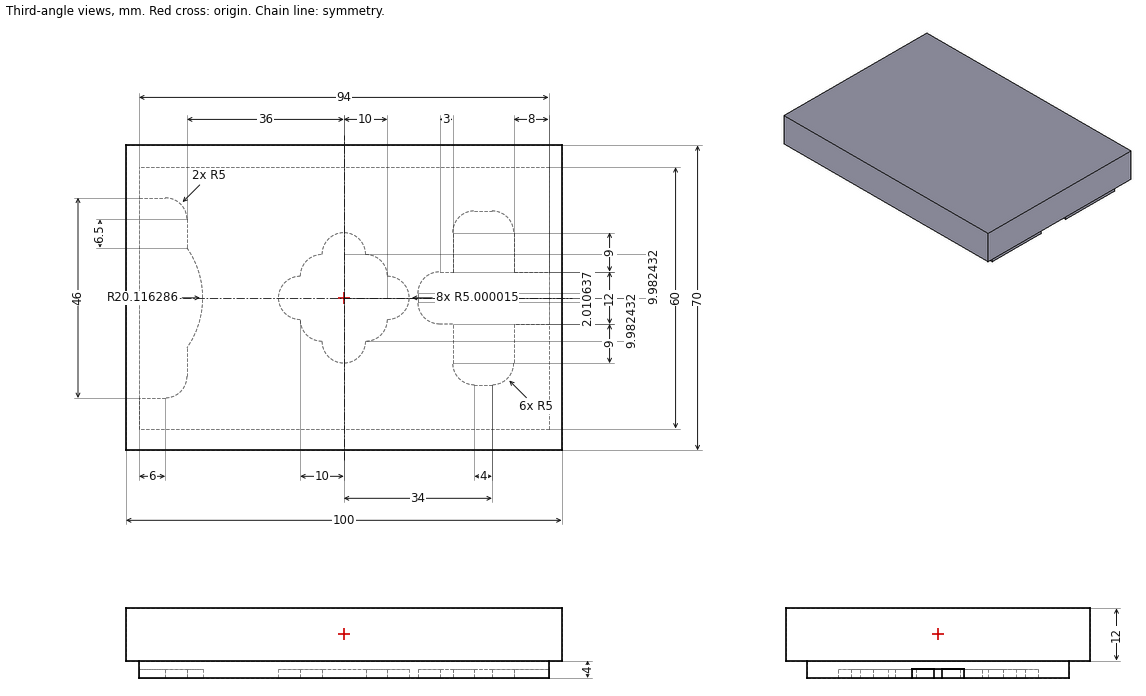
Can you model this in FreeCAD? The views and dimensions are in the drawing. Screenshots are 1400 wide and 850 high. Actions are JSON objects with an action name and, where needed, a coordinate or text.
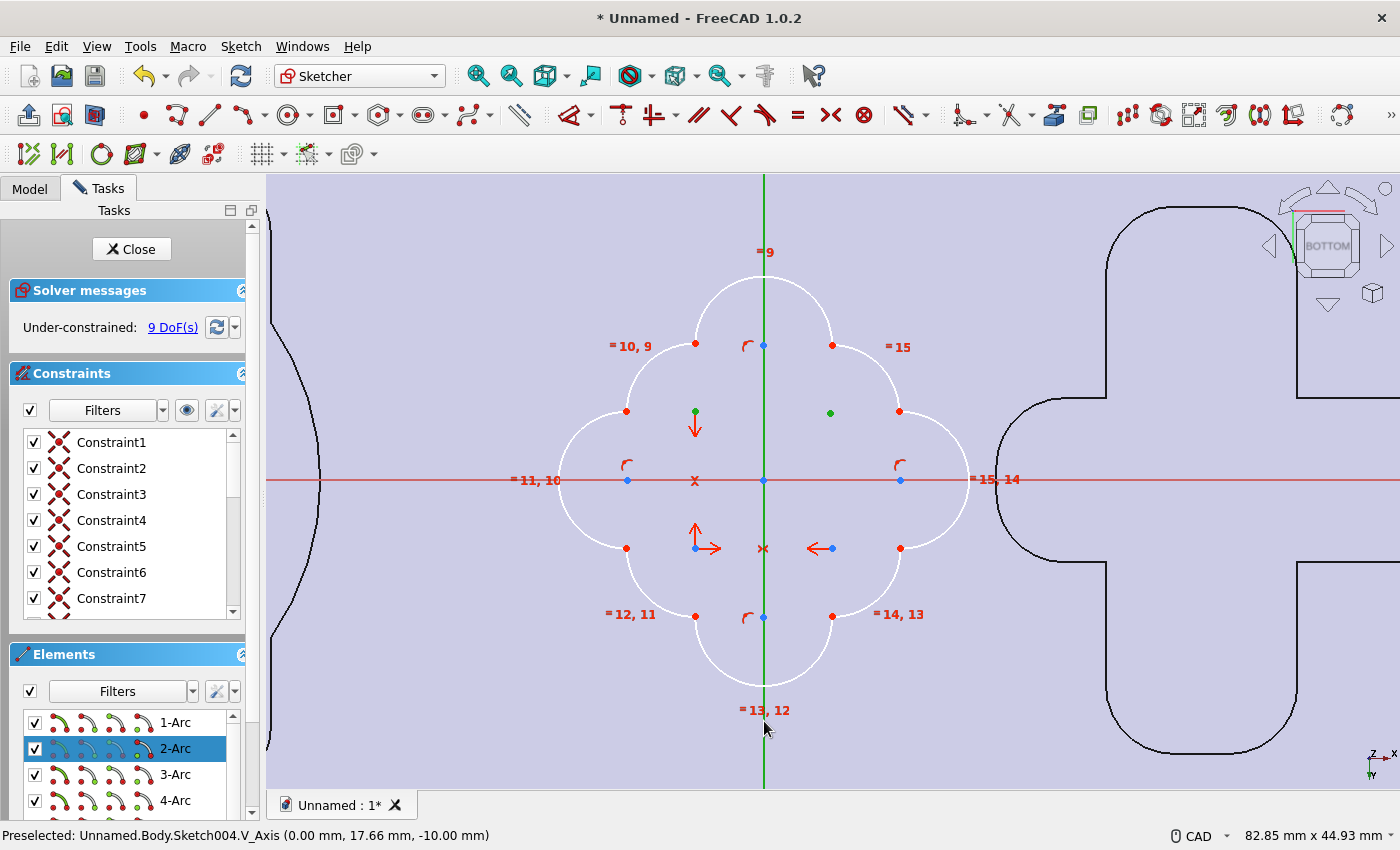
{"action": "left_click", "coordinate": [831, 116]}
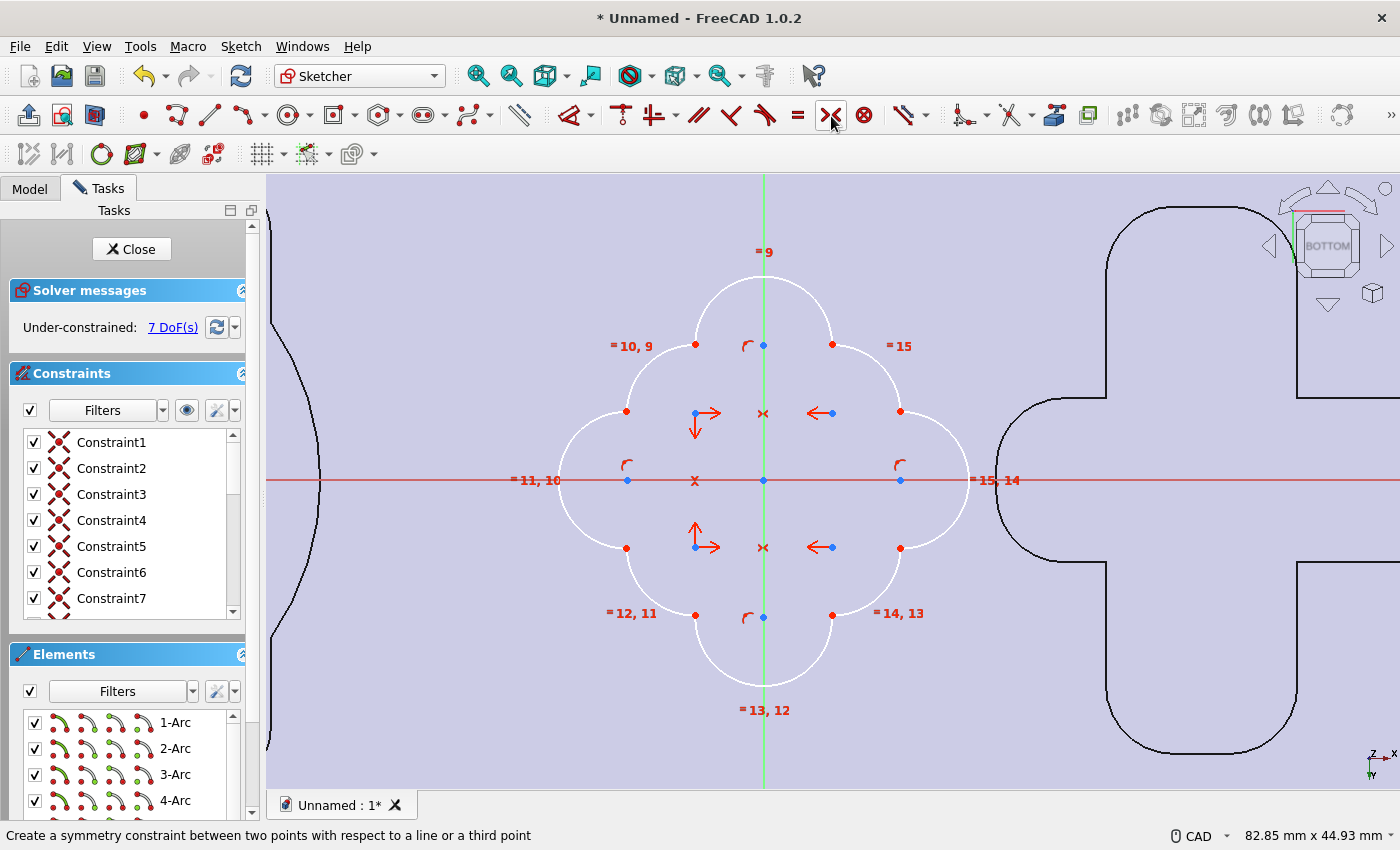
{"action": "left_click", "coordinate": [568, 116]}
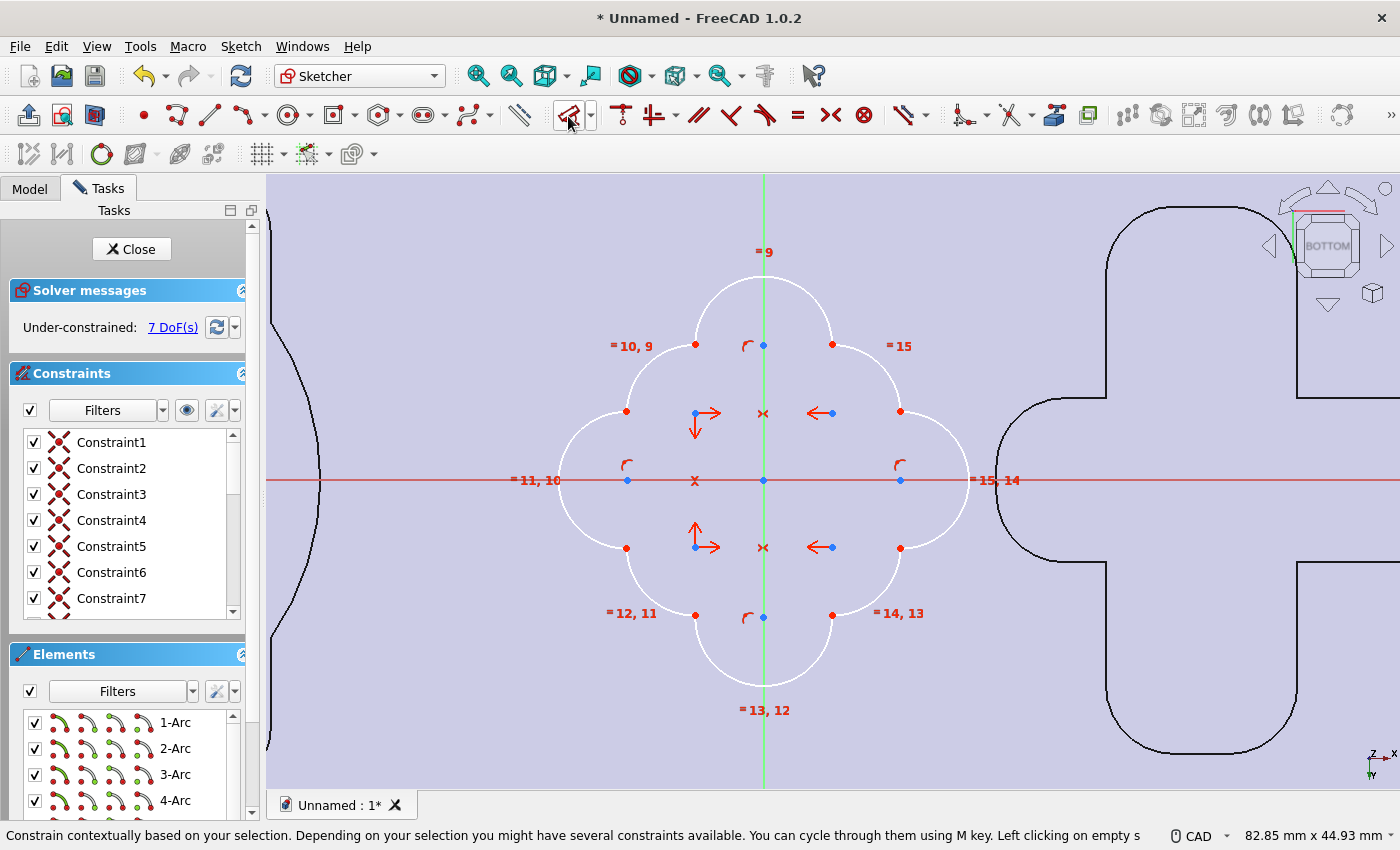
{"action": "left_click", "coordinate": [804, 290]}
{"action": "left_click", "coordinate": [823, 264]}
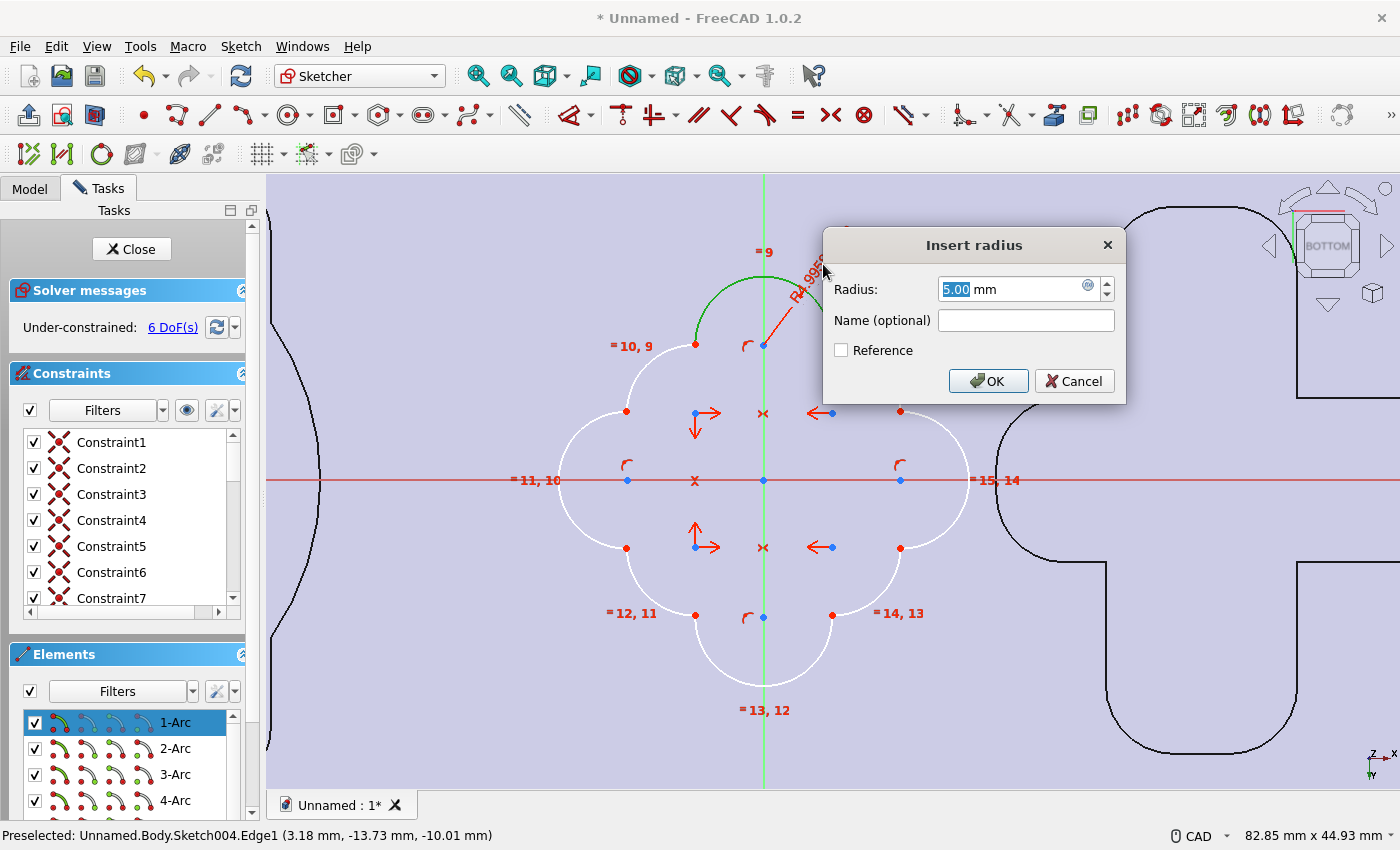
{"action": "type", "text": "5.000015"}
{"action": "key", "text": "Return"}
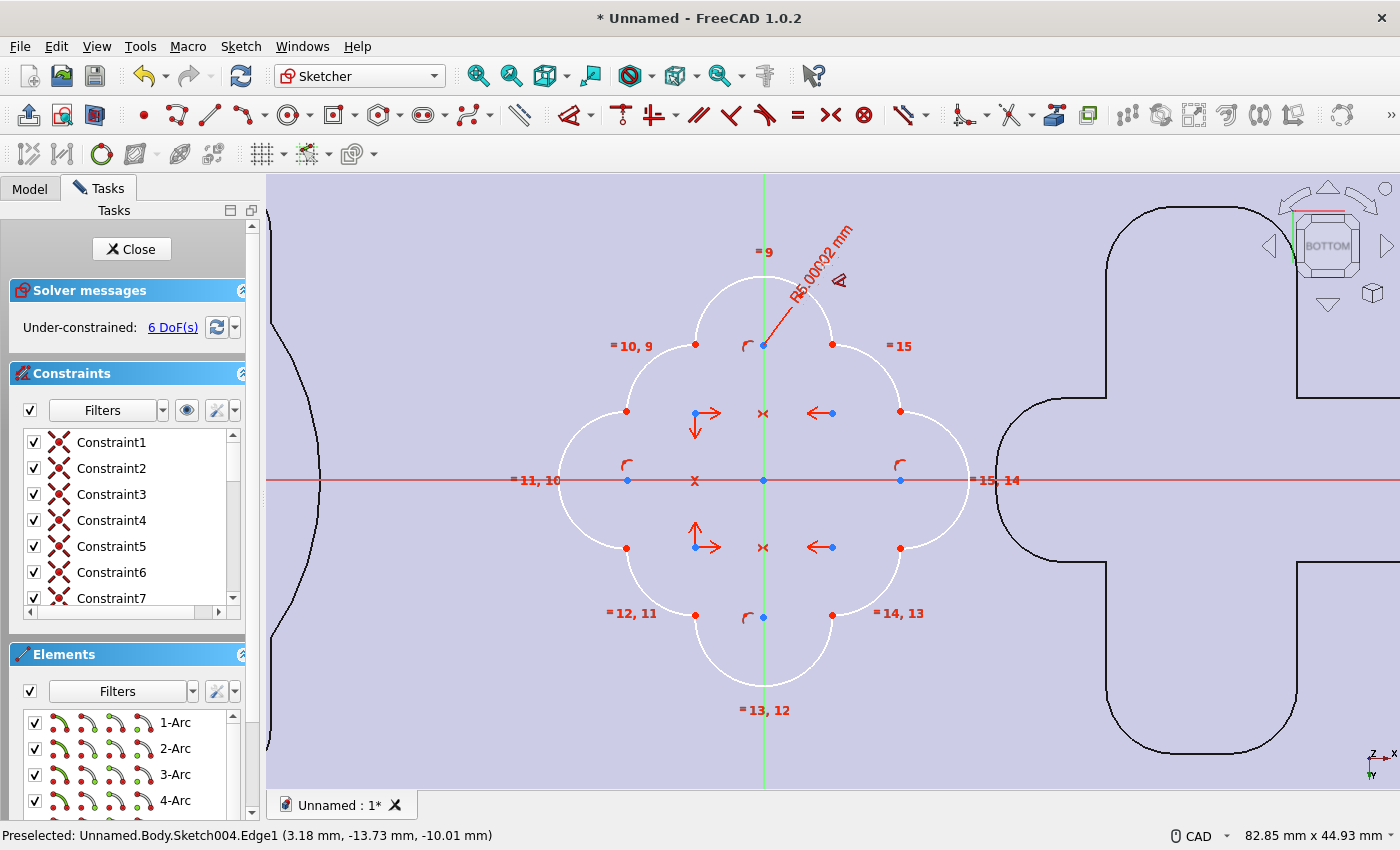
{"action": "left_click", "coordinate": [627, 412]}
{"action": "left_click", "coordinate": [695, 378]}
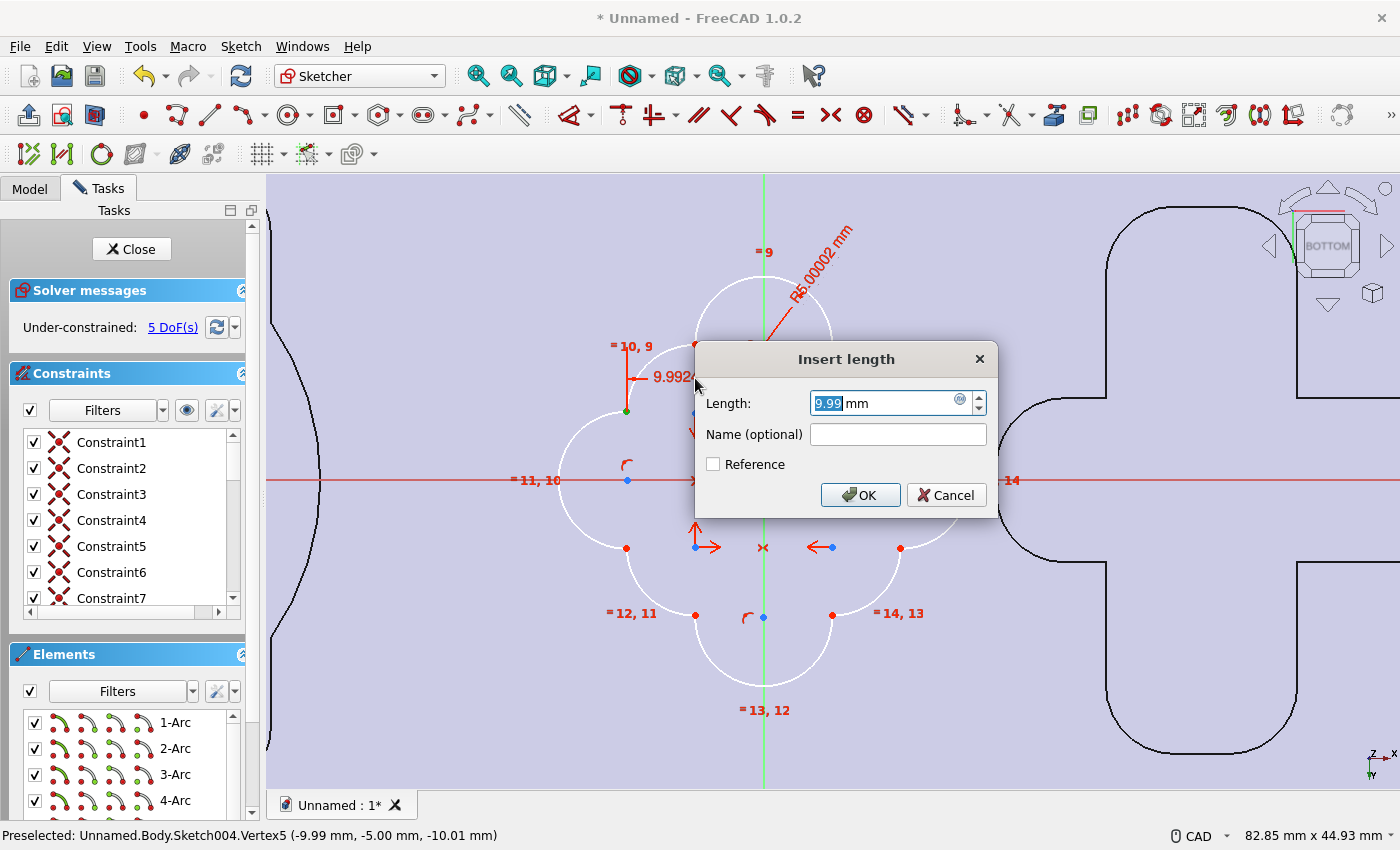
{"action": "type", "text": "10"}
{"action": "key", "text": "Return"}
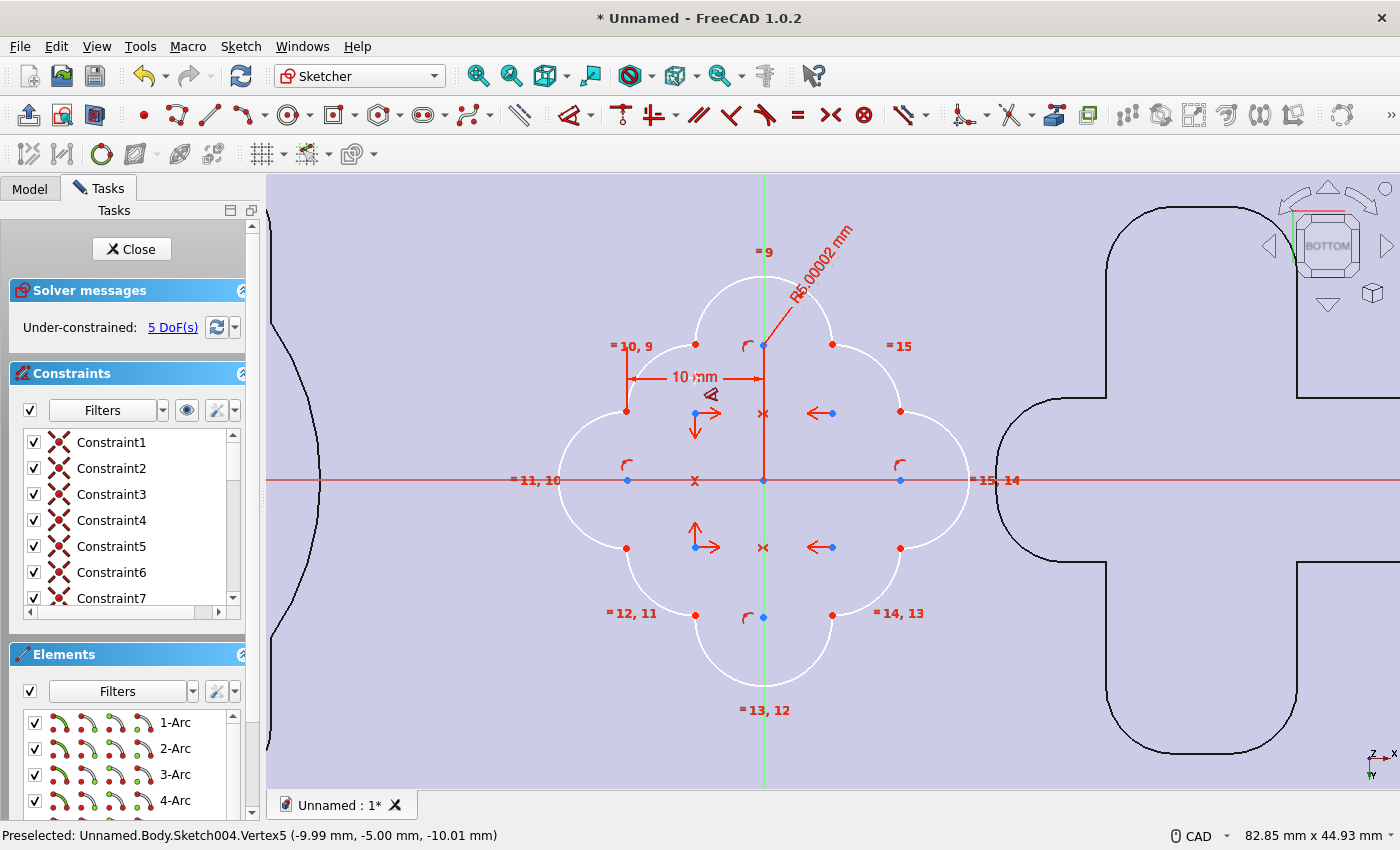
{"action": "left_click", "coordinate": [627, 480]}
{"action": "left_click", "coordinate": [695, 514]}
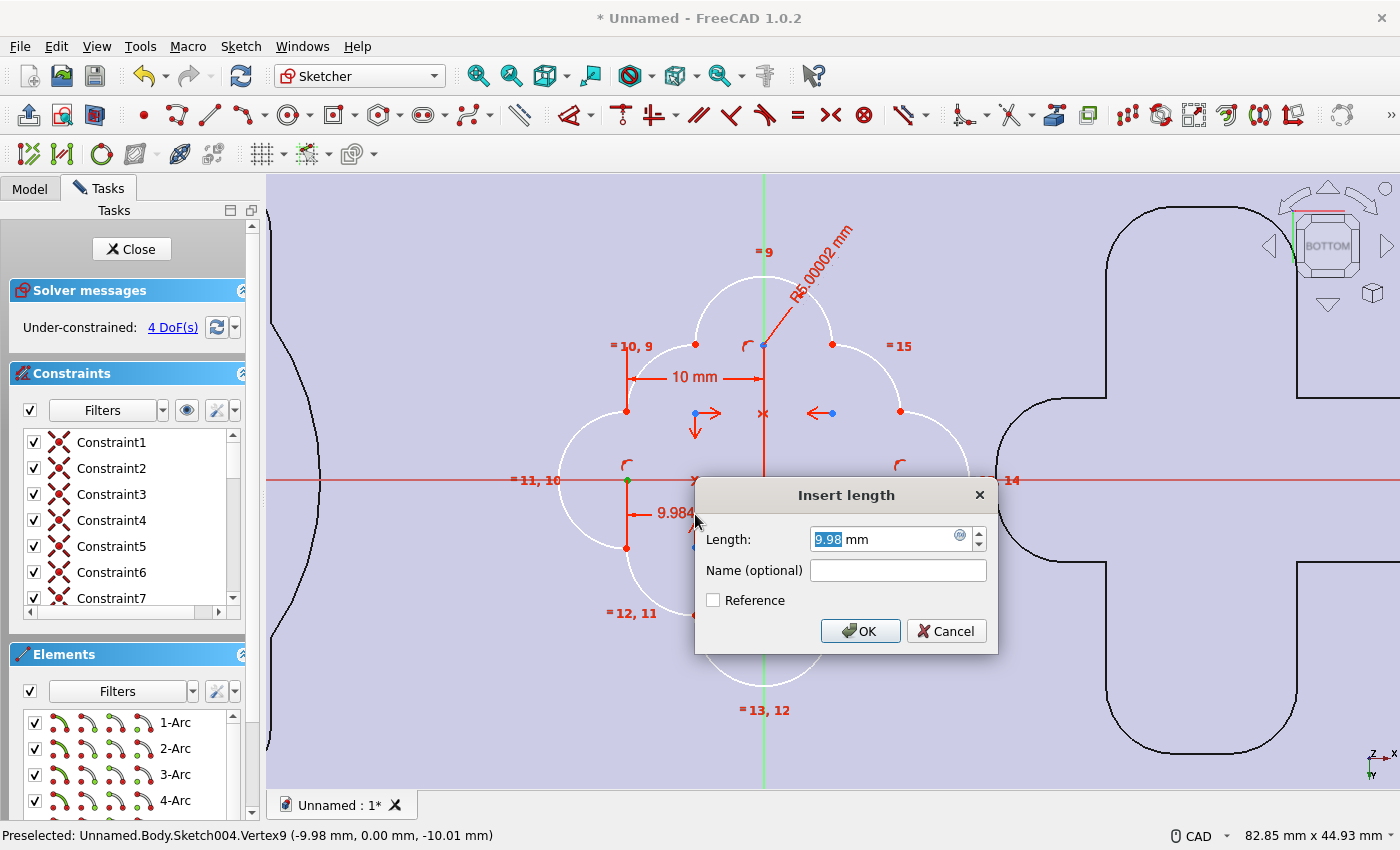
{"action": "type", "text": "10"}
{"action": "key", "text": "Return"}